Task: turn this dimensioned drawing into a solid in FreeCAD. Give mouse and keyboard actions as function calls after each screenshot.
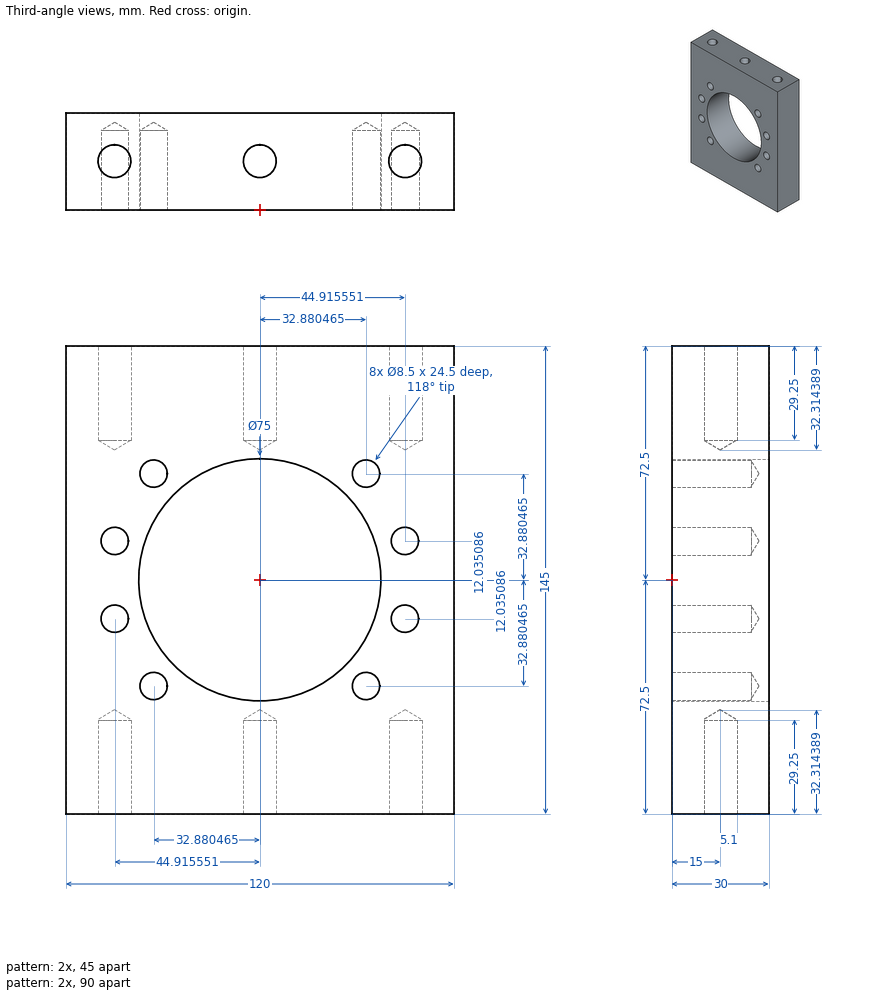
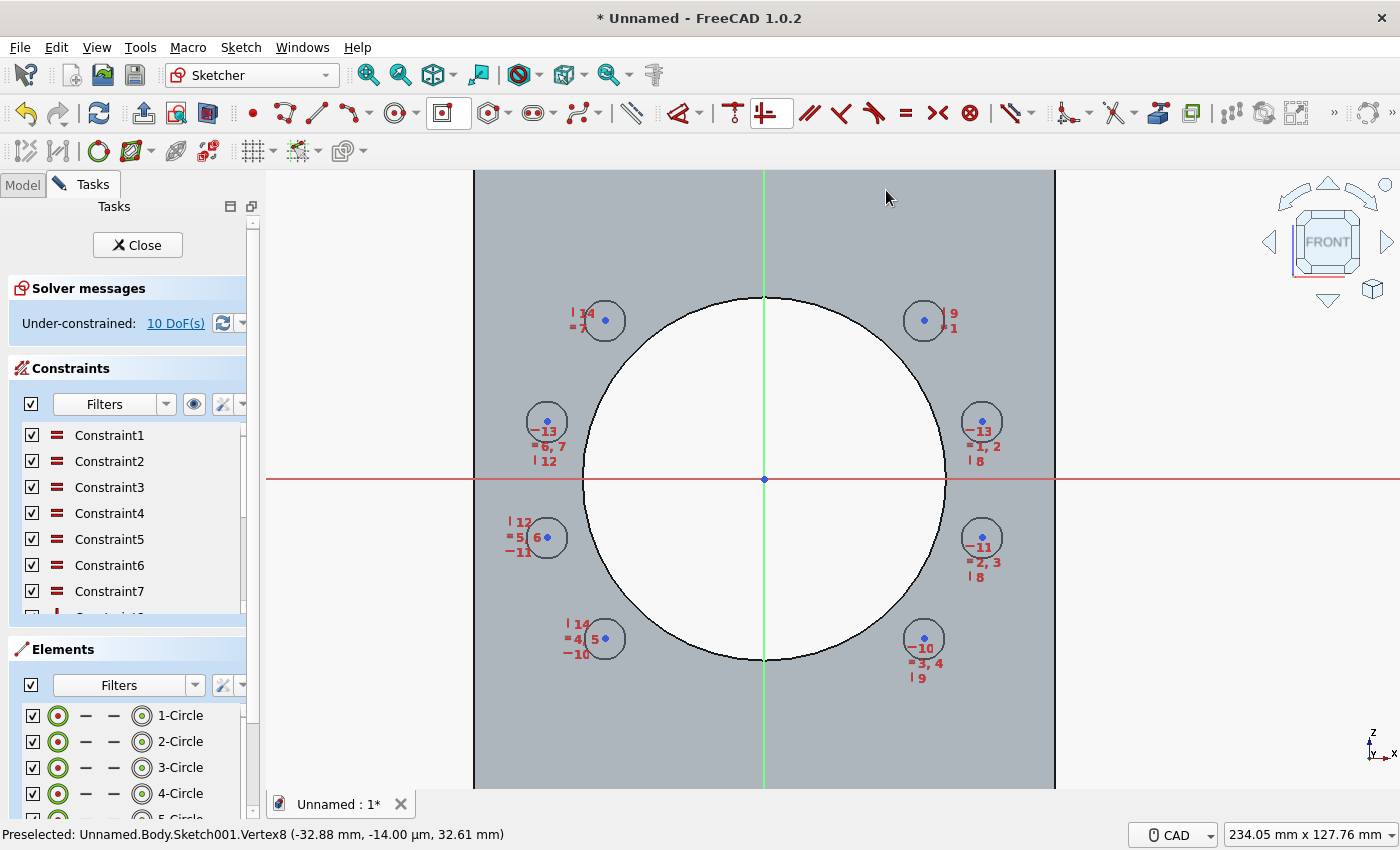
click(924, 321)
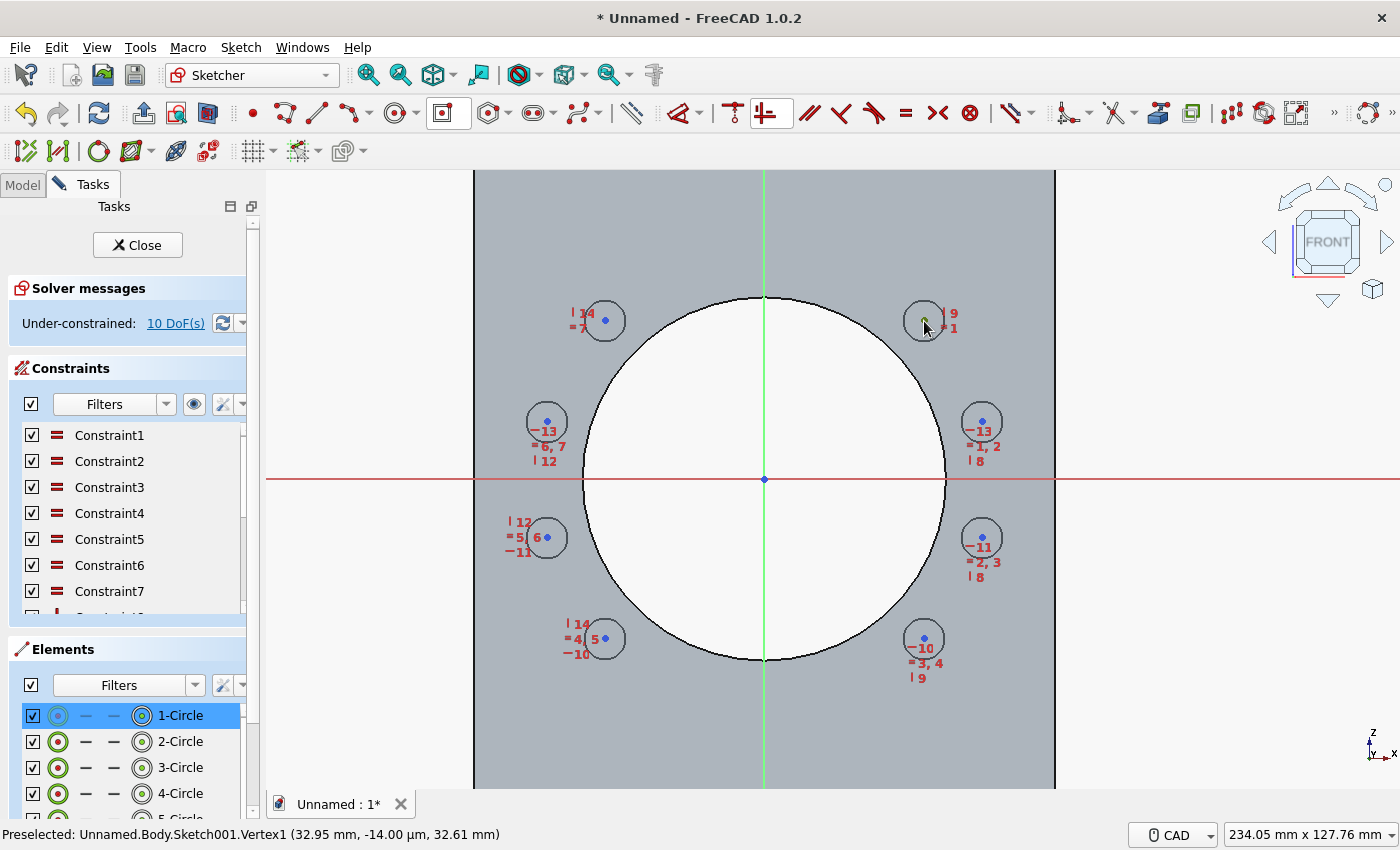
click(605, 321)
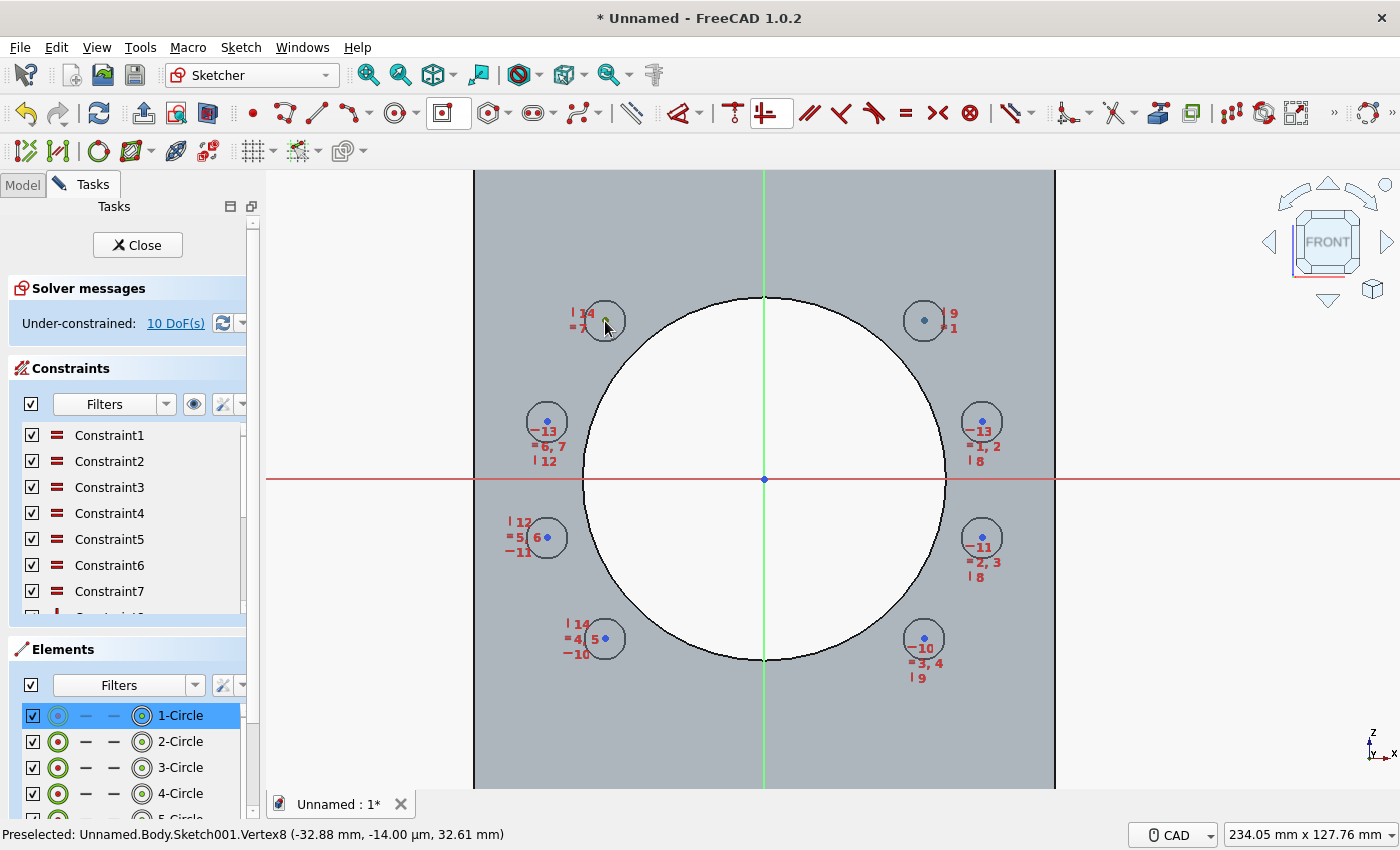
key(h)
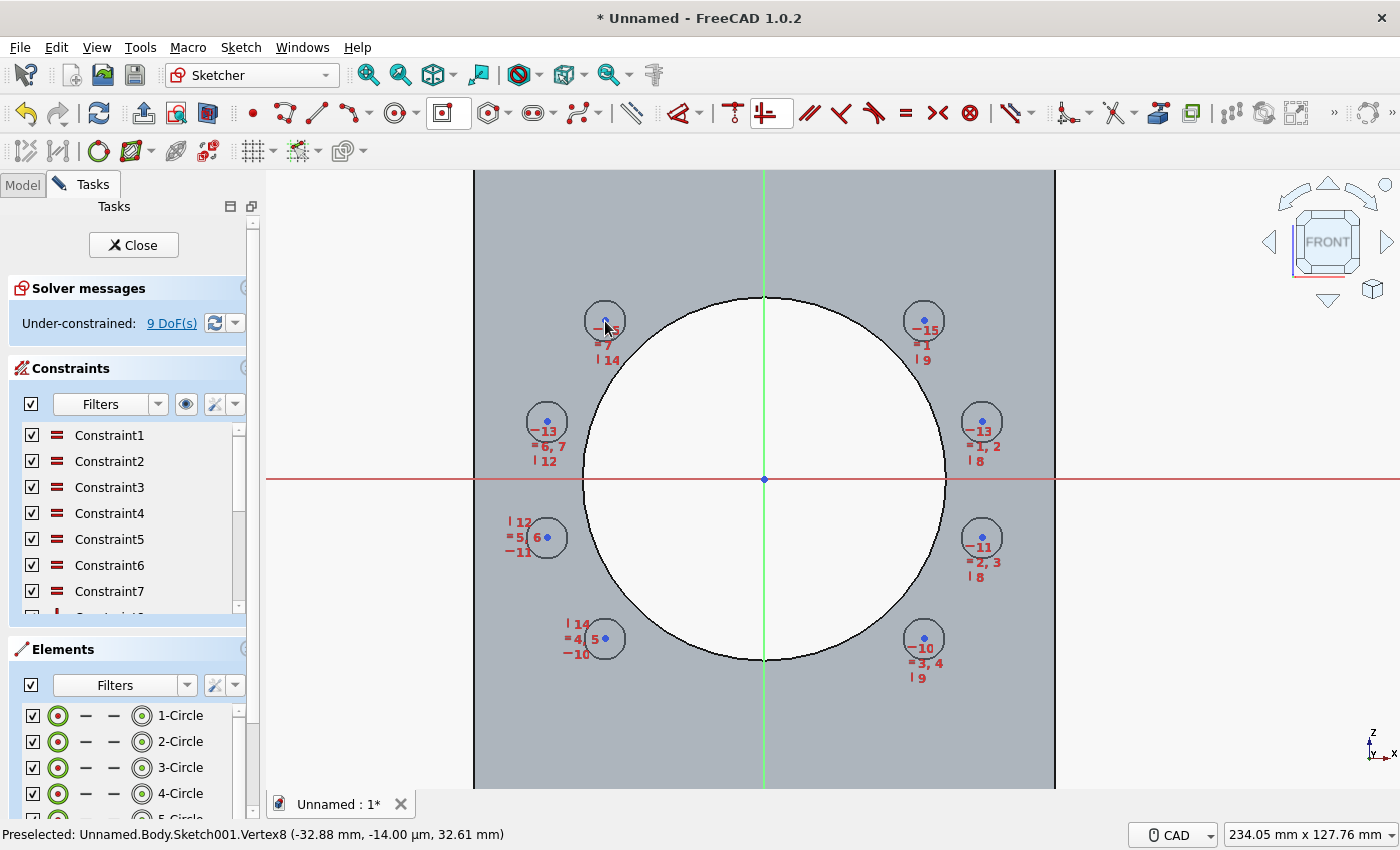
click(678, 114)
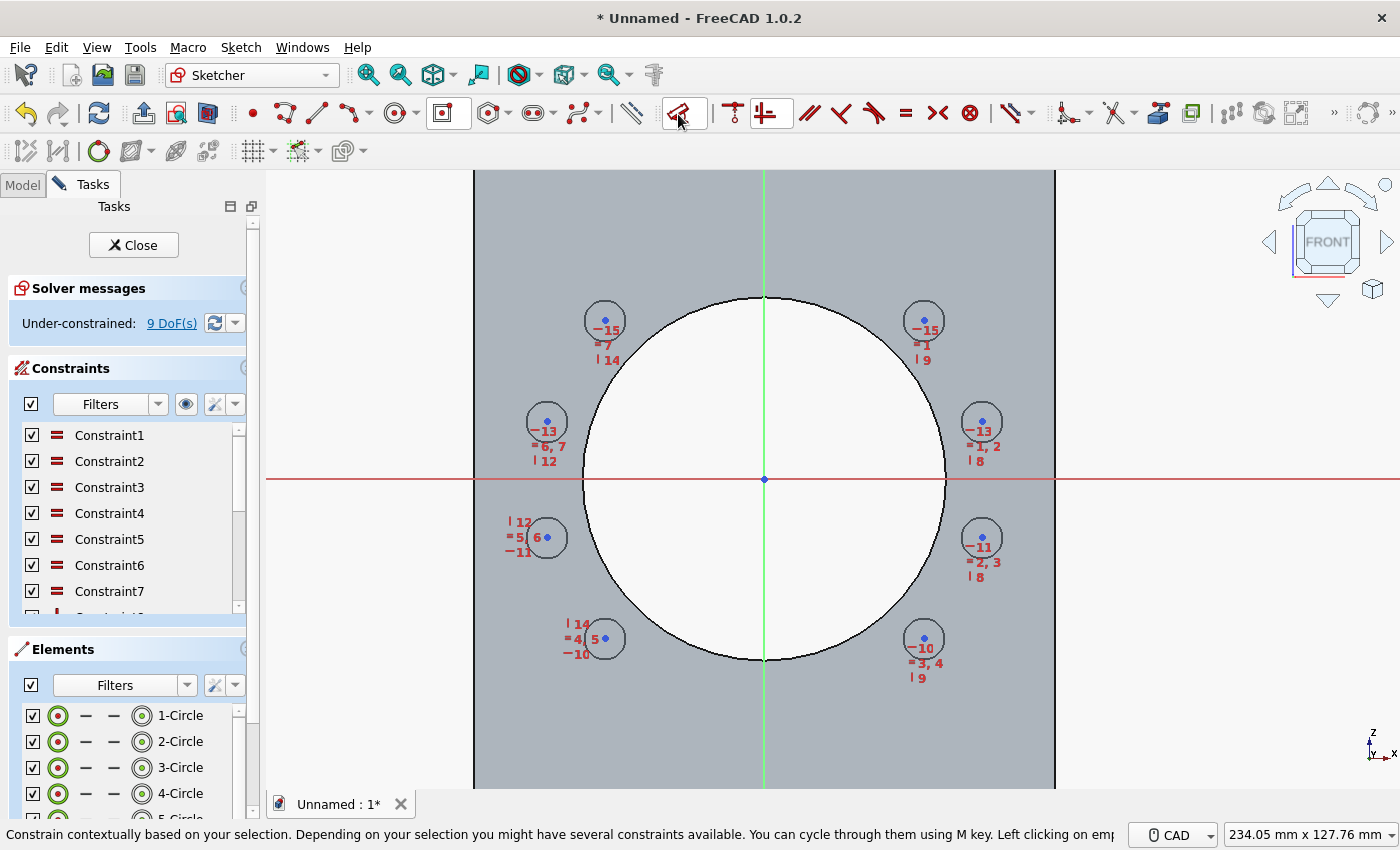
click(938, 306)
click(960, 283)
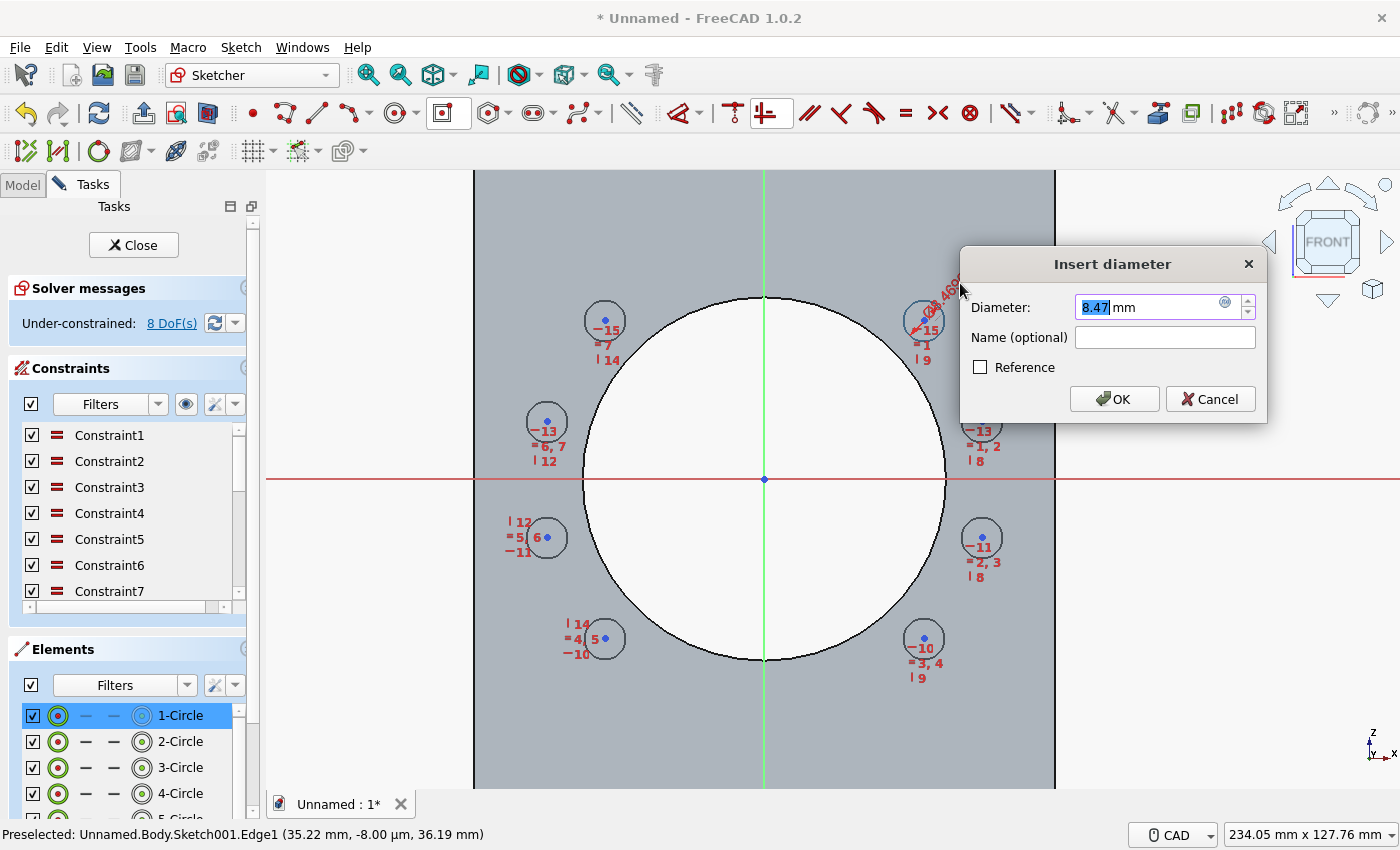
text(8.5)
key(Return)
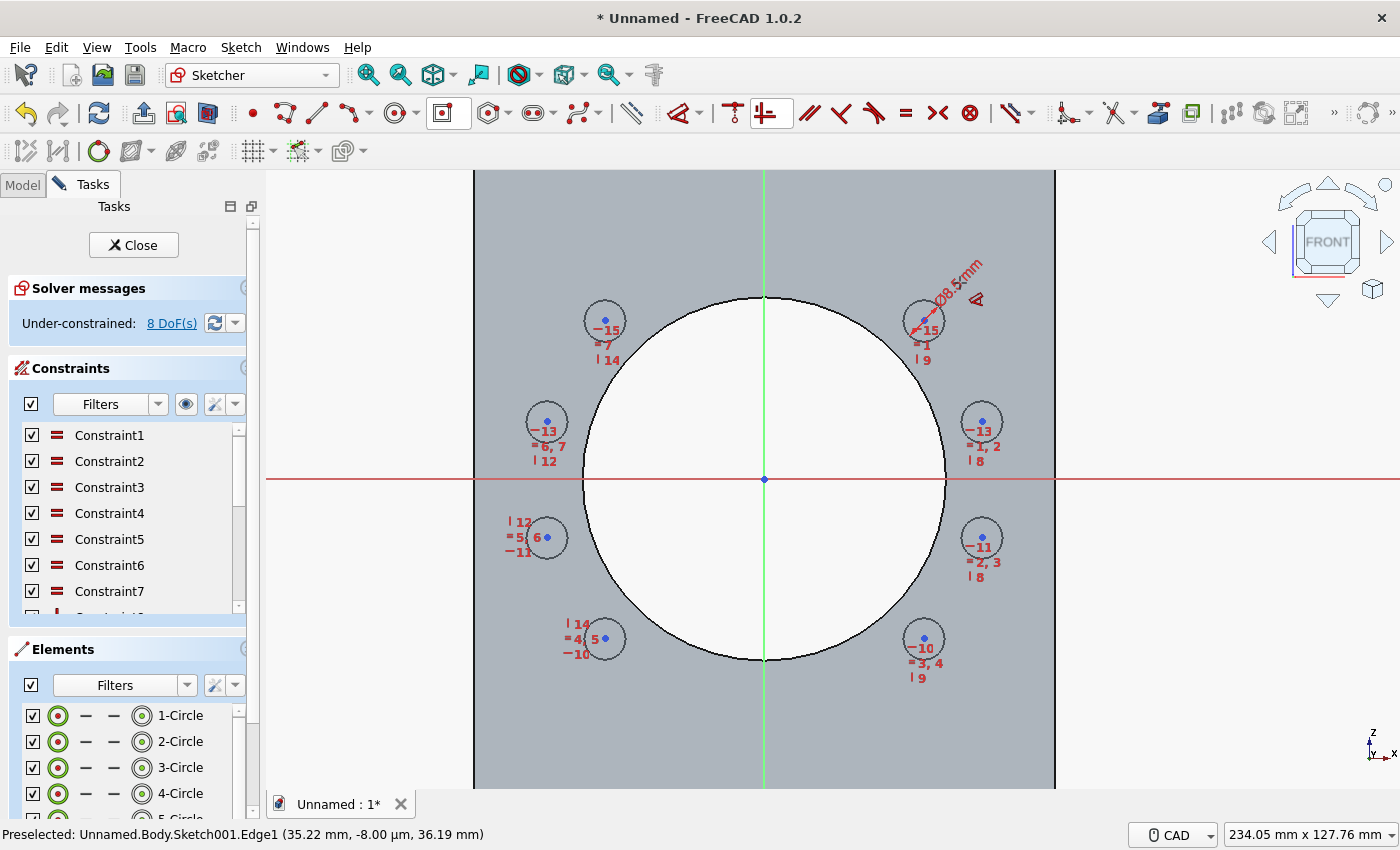
click(924, 321)
click(844, 287)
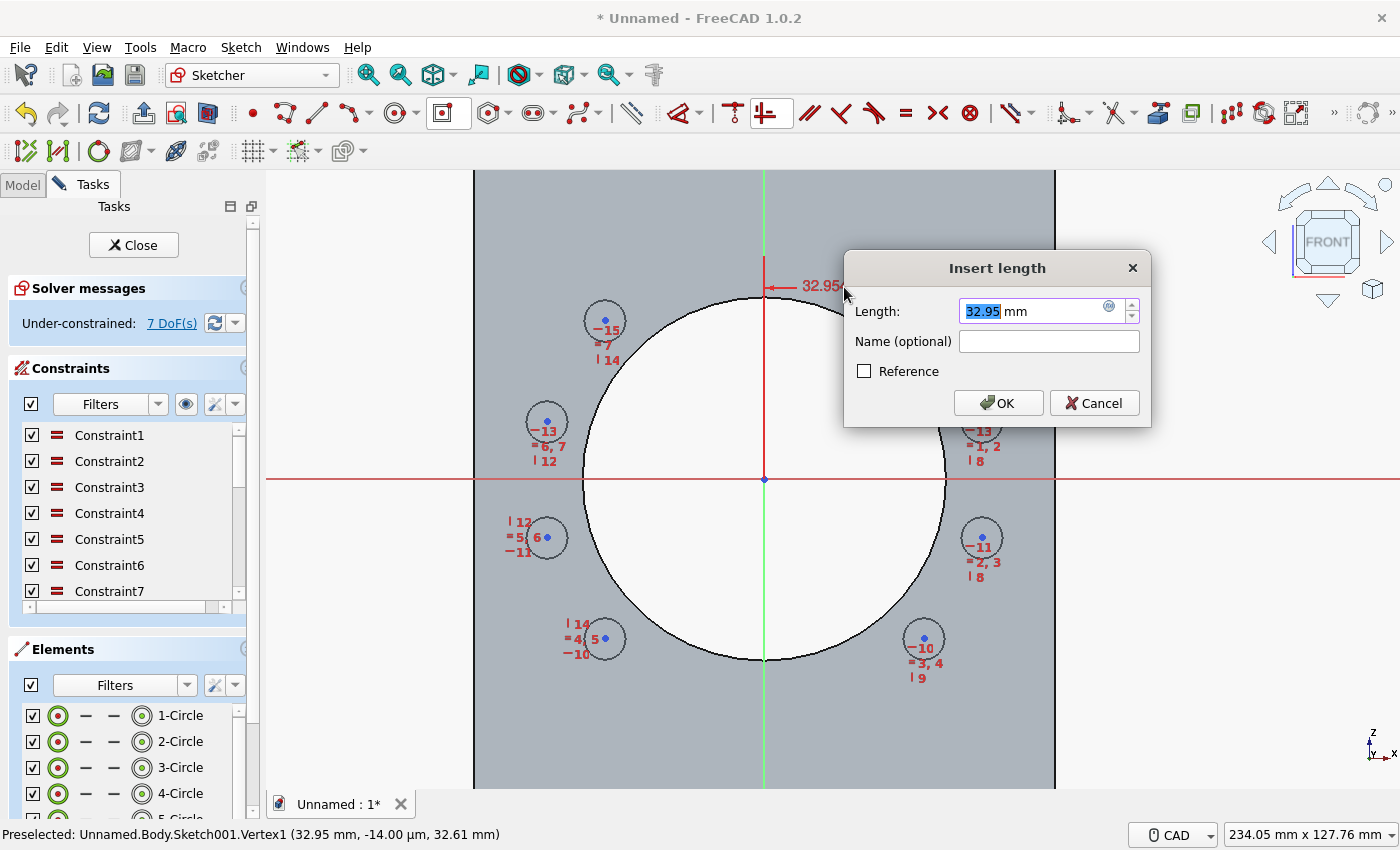
text(32.880465)
key(Return)